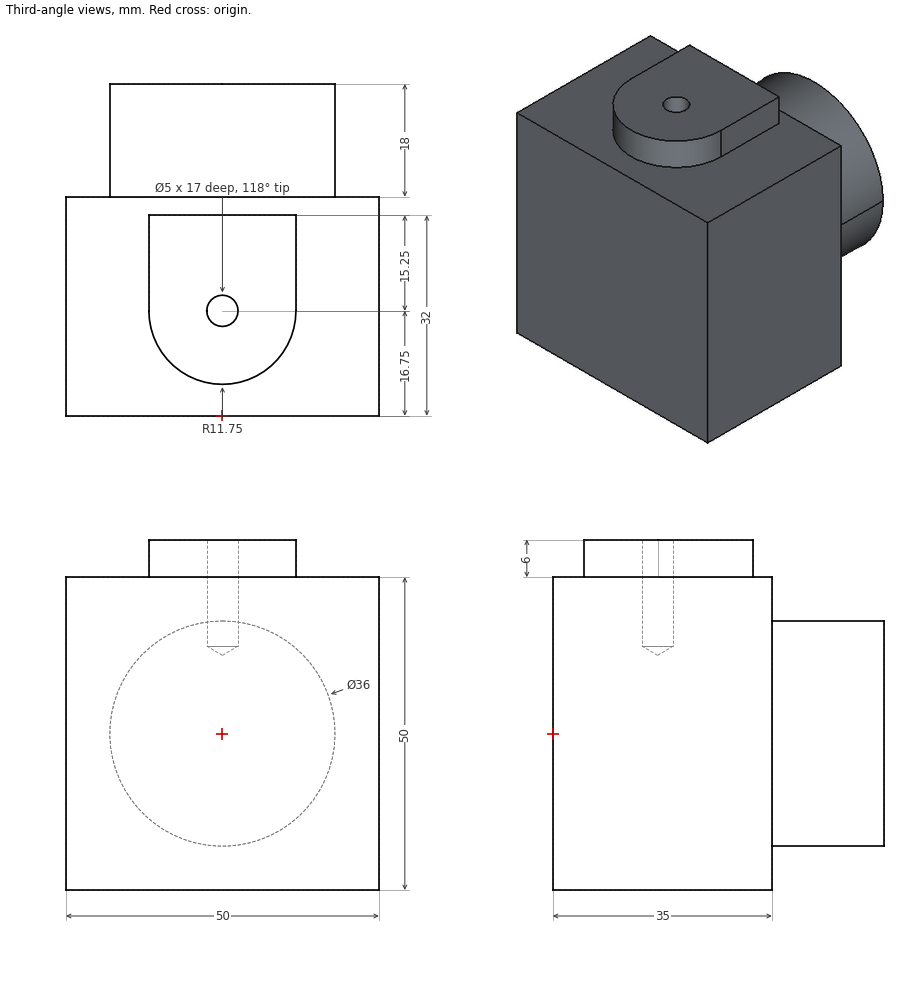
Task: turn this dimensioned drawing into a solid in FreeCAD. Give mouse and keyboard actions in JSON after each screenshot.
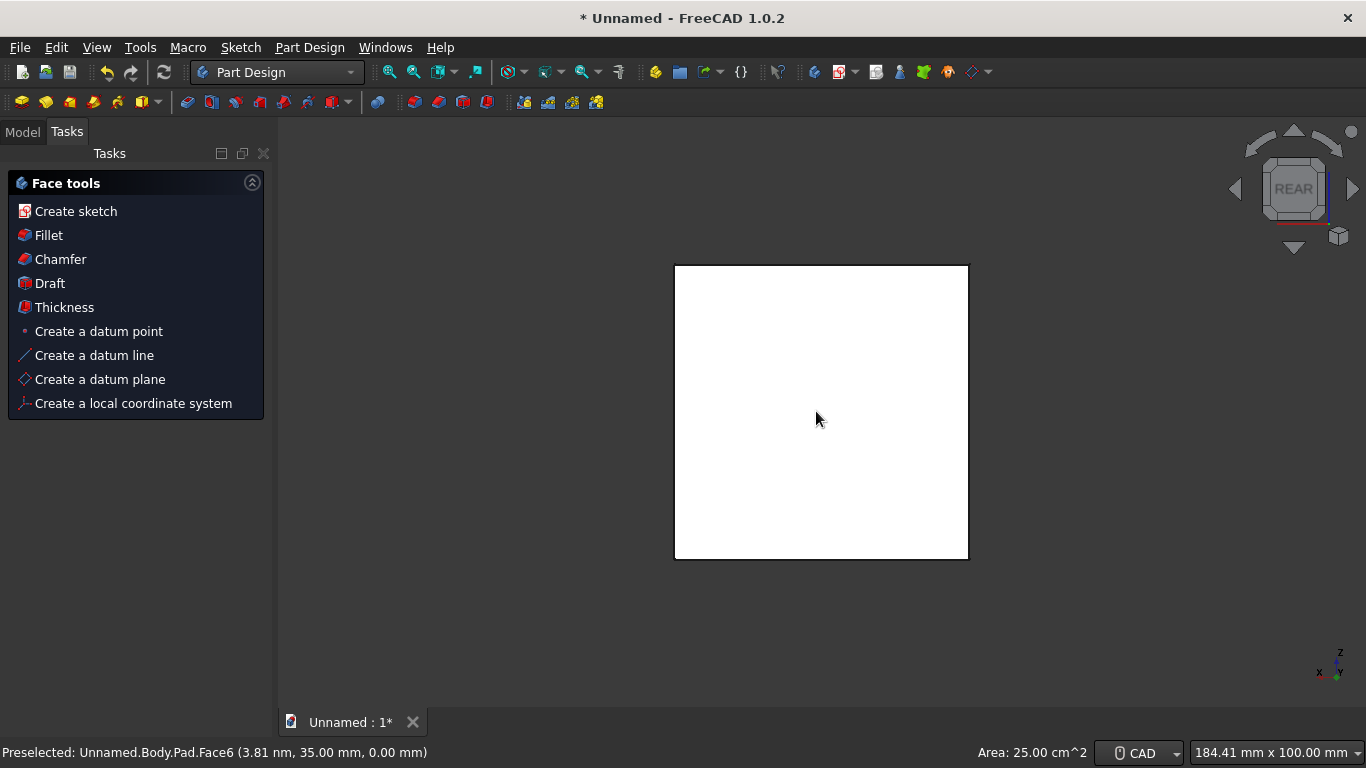
{"action": "left_click", "coordinate": [840, 72]}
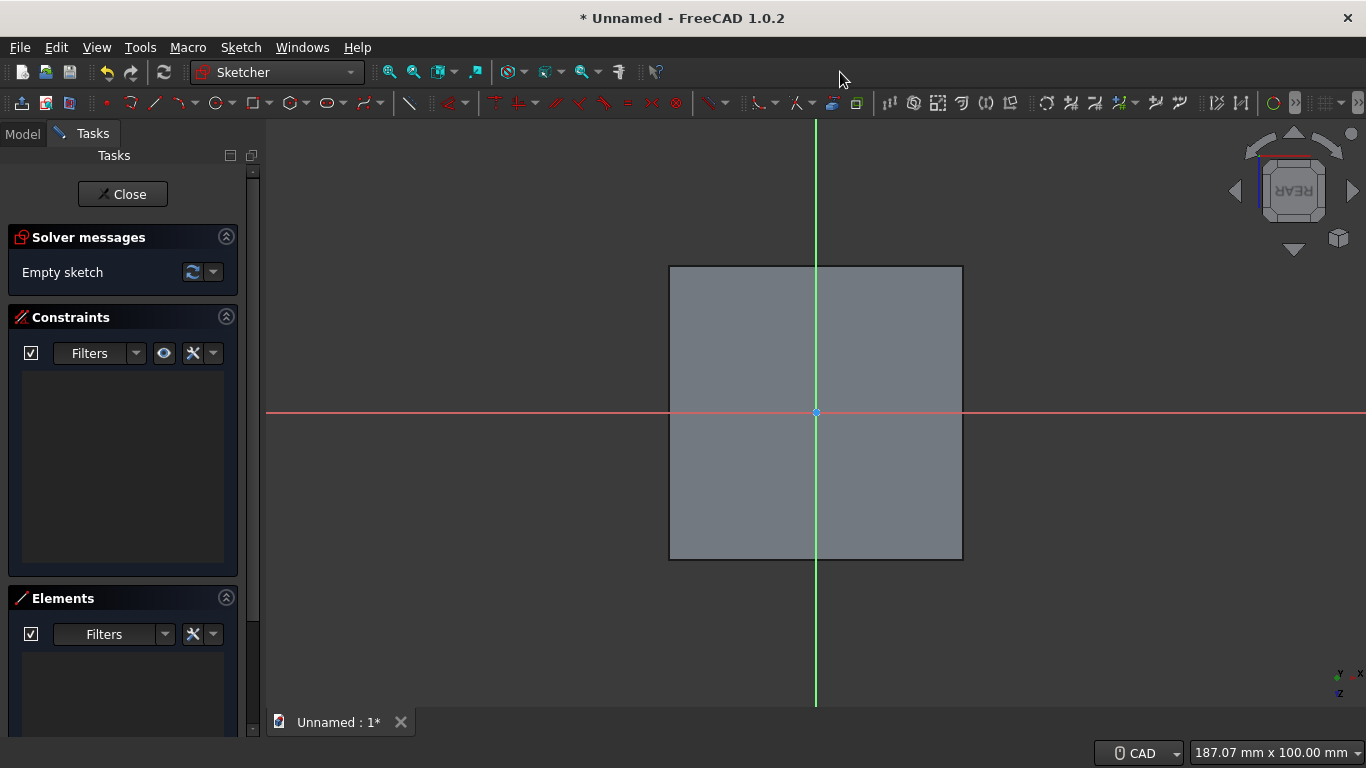
{"action": "scroll", "coordinate": [899, 413], "scroll_direction": "up", "scroll_amount": 3}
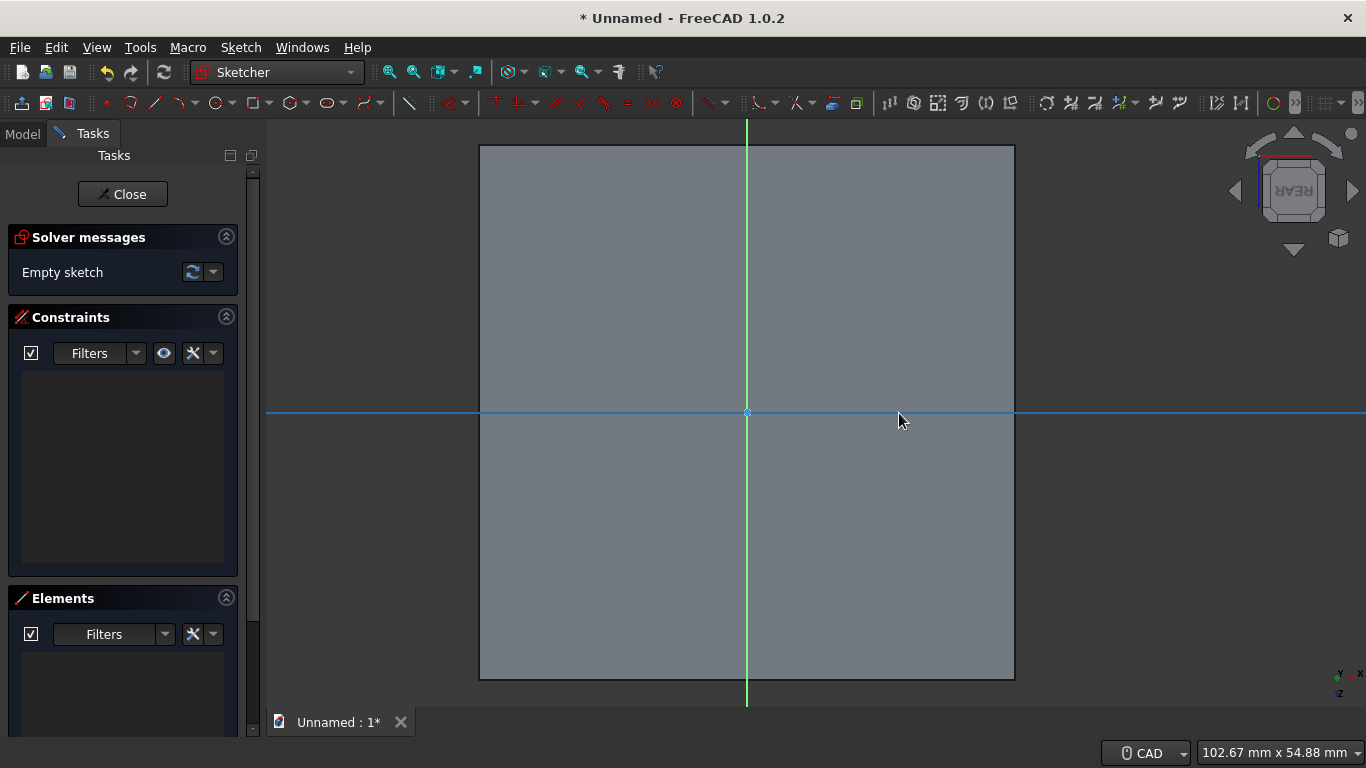
{"action": "key", "text": "g c"}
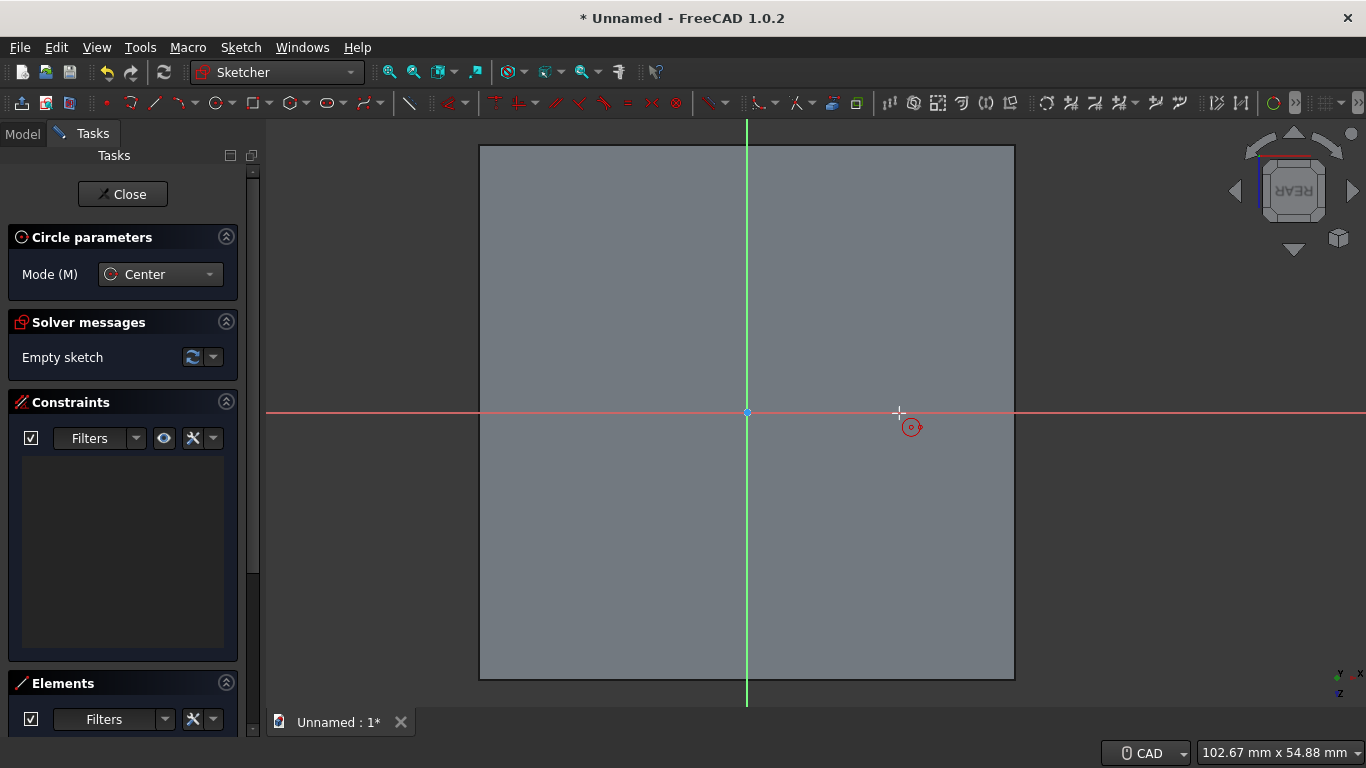
{"action": "left_click", "coordinate": [747, 413]}
{"action": "left_click", "coordinate": [884, 276]}
{"action": "key", "text": "Escape"}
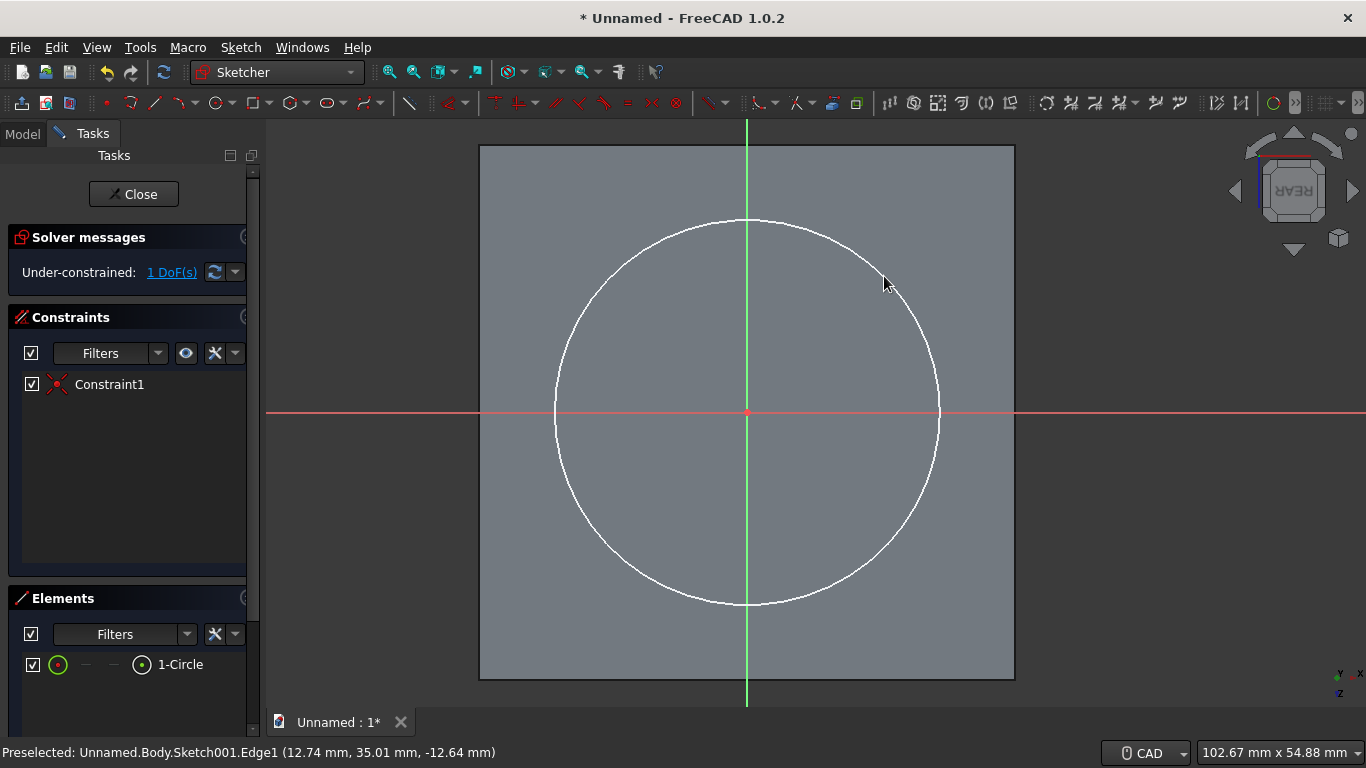
{"action": "key", "text": "d"}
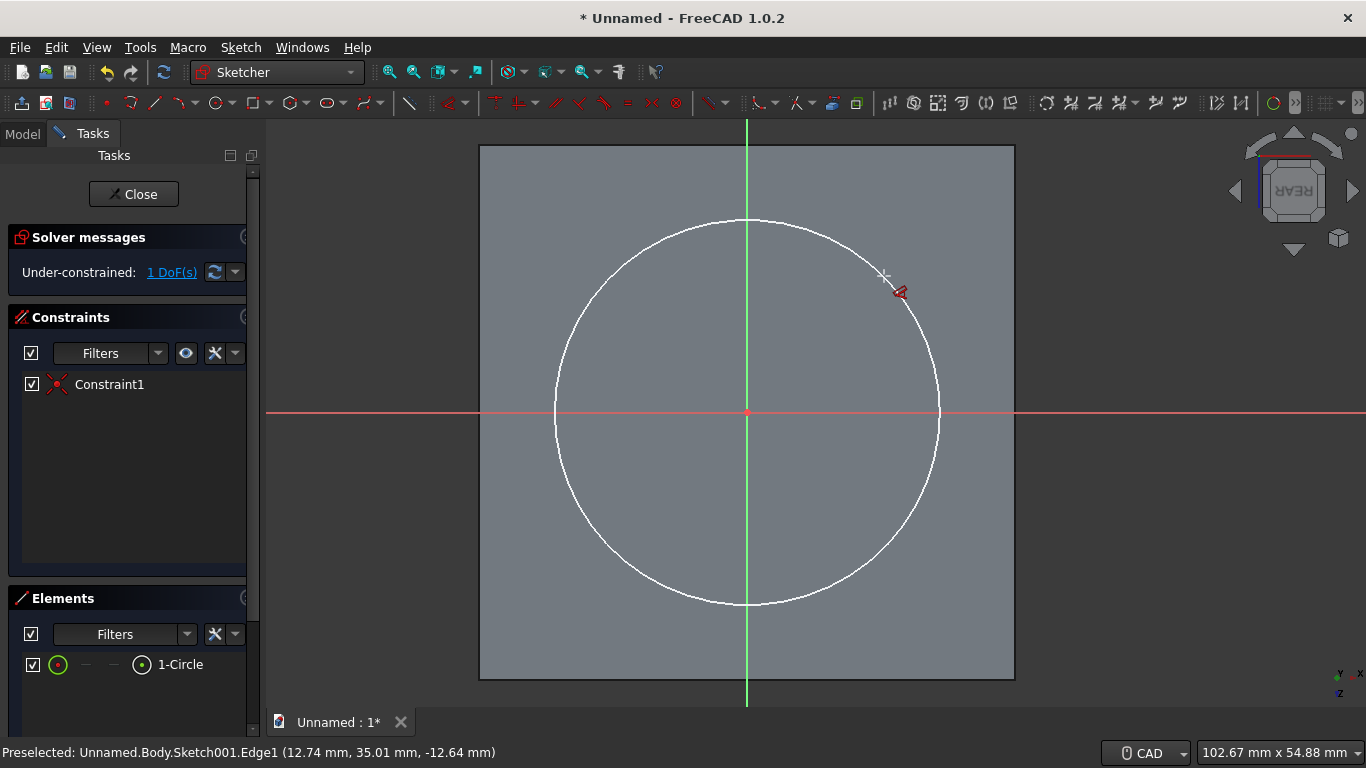
{"action": "left_click", "coordinate": [883, 276]}
{"action": "left_click", "coordinate": [906, 253]}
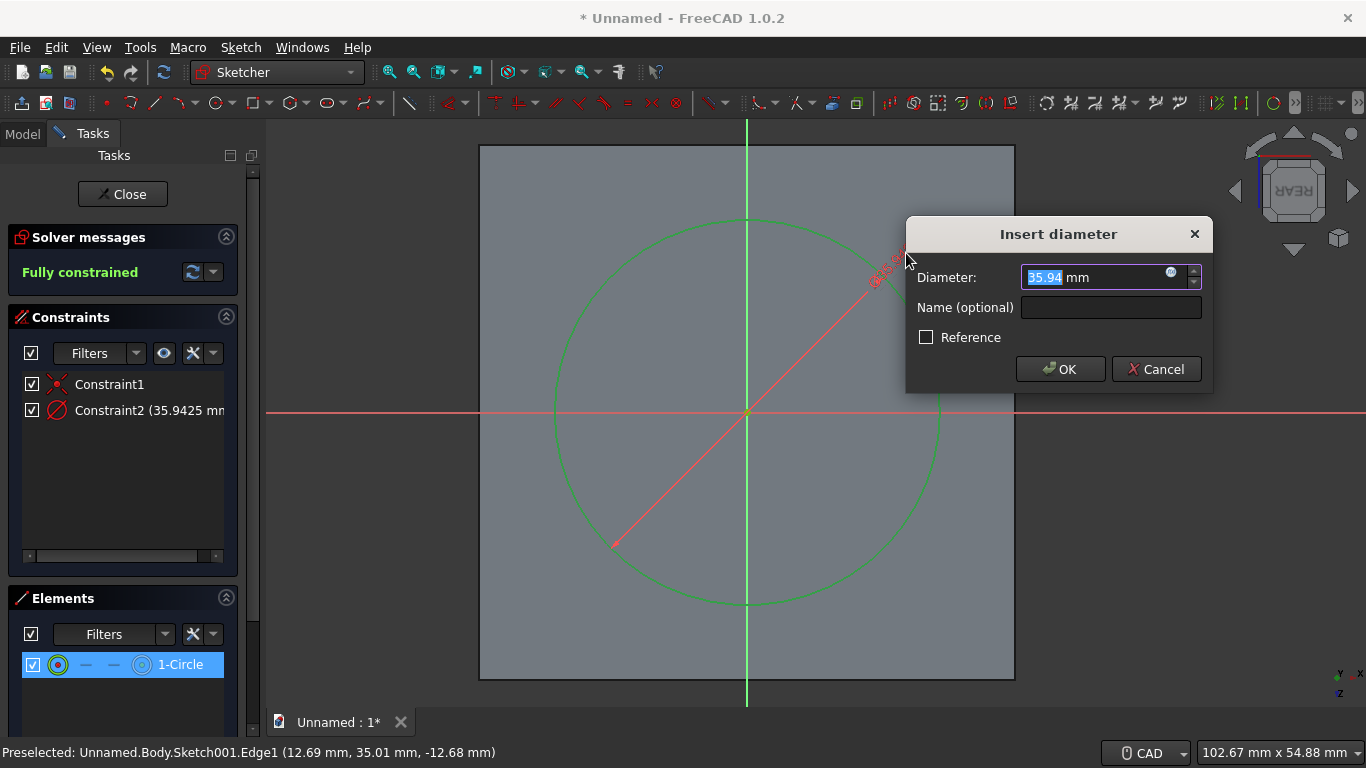
{"action": "type", "text": "36"}
{"action": "key", "text": "Return"}
{"action": "key", "text": "Escape"}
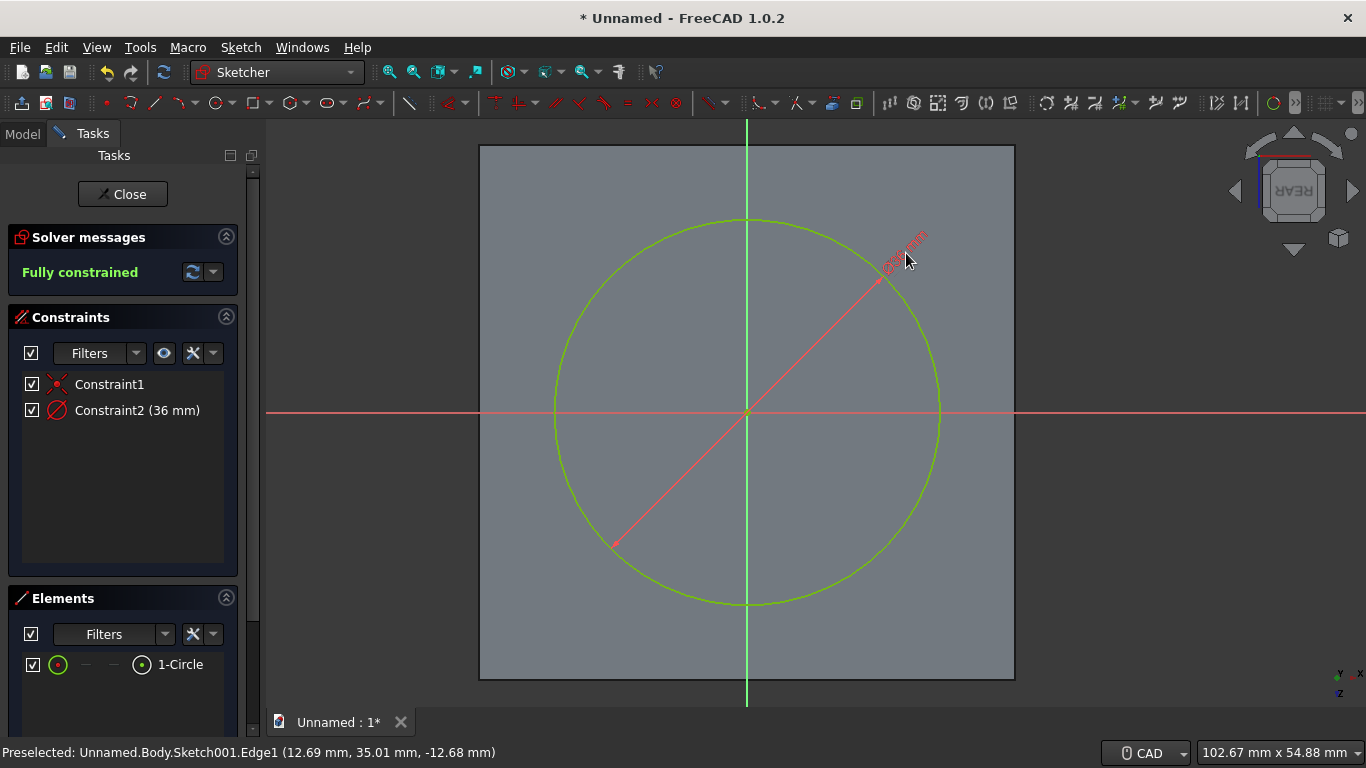
{"action": "left_click", "coordinate": [123, 194]}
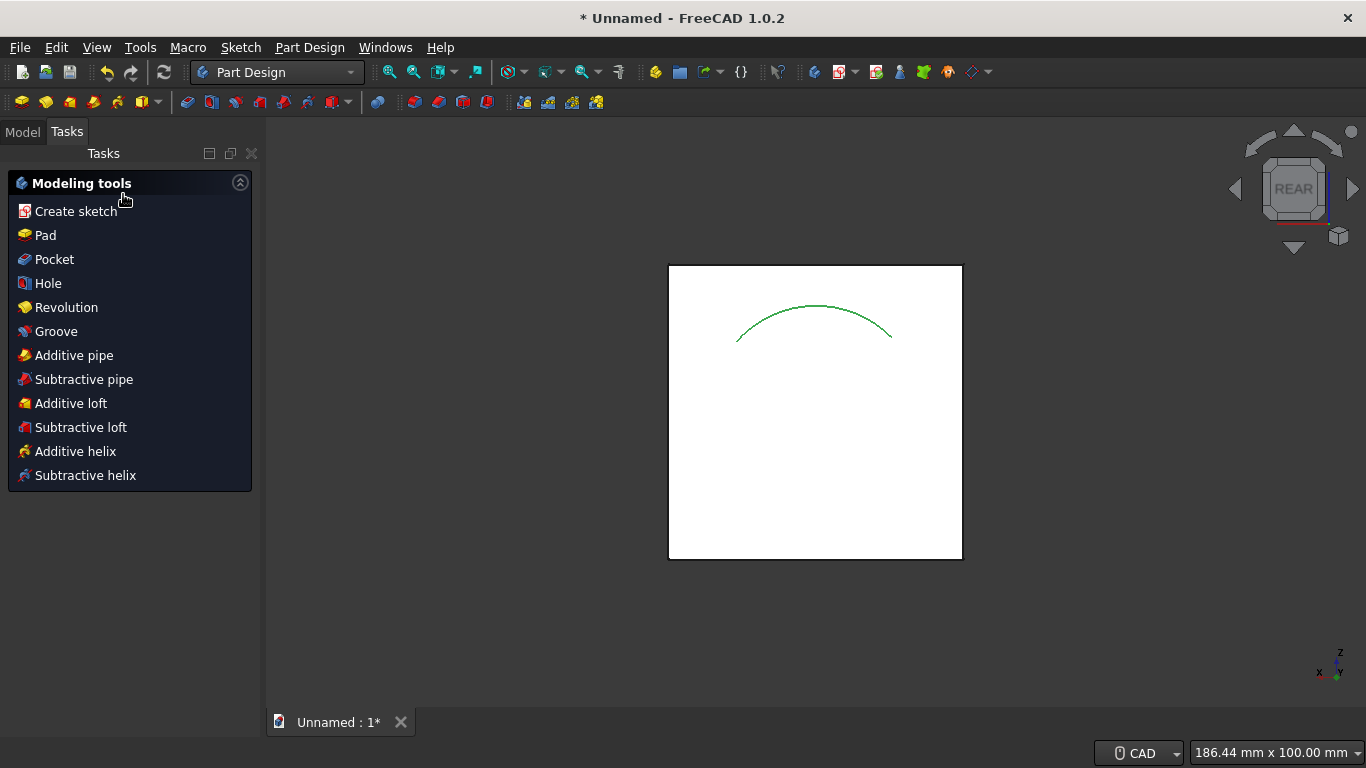
{"action": "left_click", "coordinate": [22, 102]}